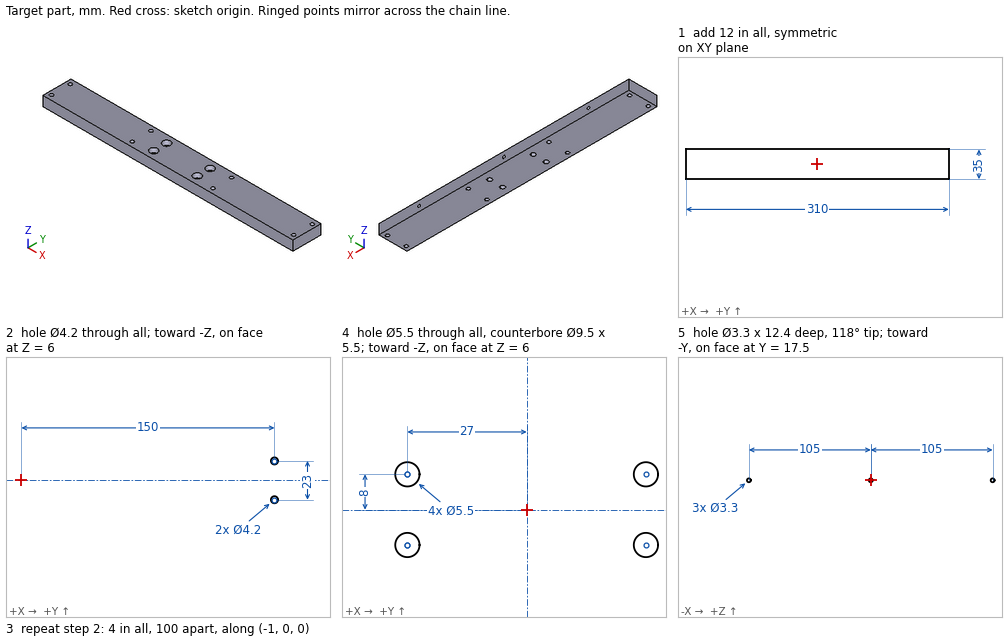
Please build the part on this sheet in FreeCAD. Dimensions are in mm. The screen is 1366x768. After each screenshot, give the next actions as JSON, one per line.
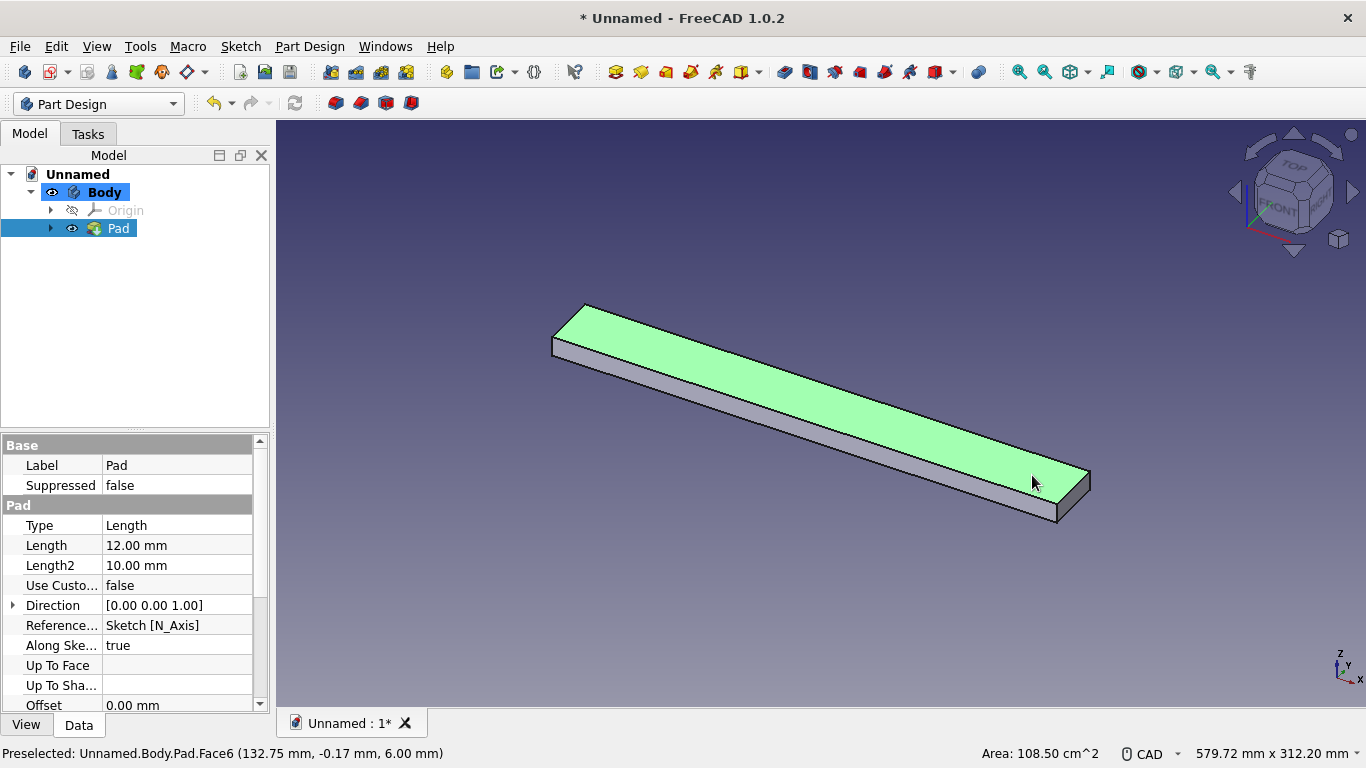
{"action": "left_click", "coordinate": [50, 72]}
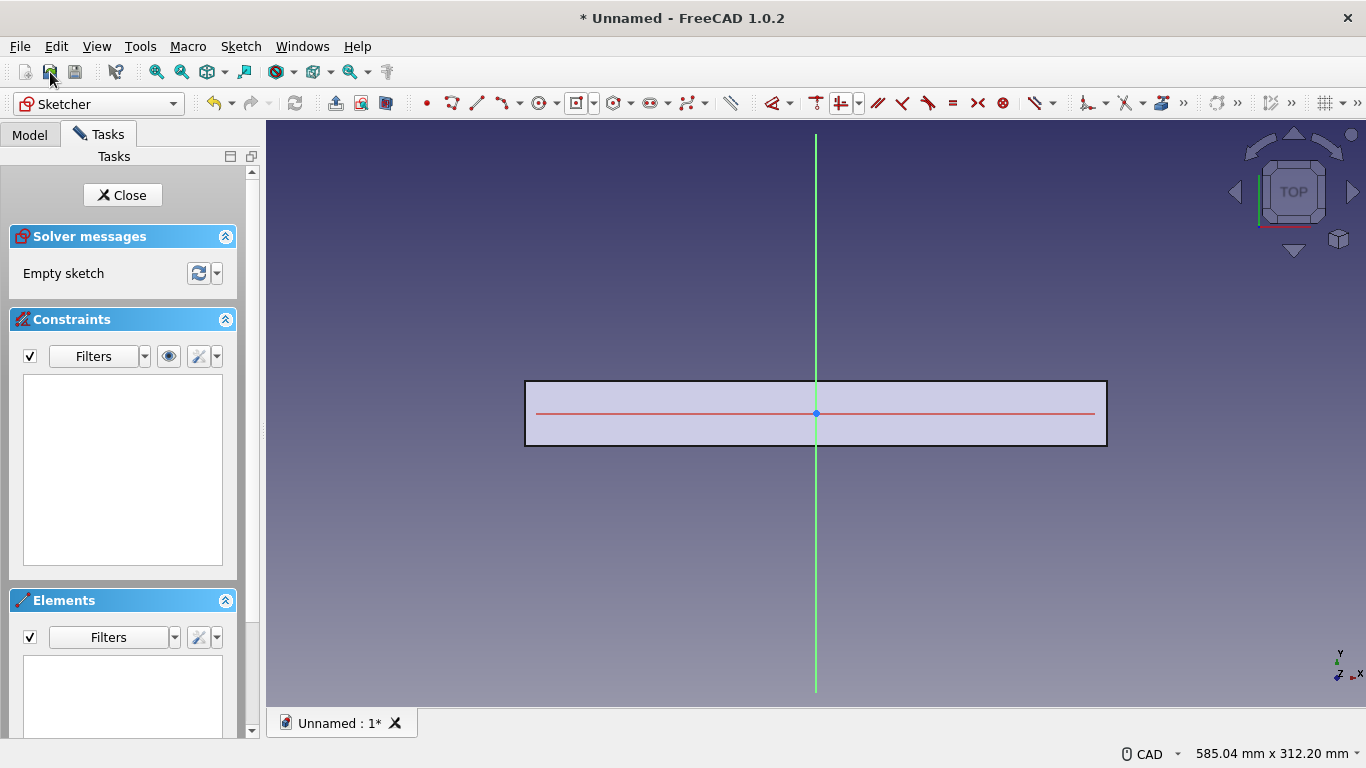
{"action": "scroll", "coordinate": [1153, 414], "scroll_direction": "up", "scroll_amount": 10}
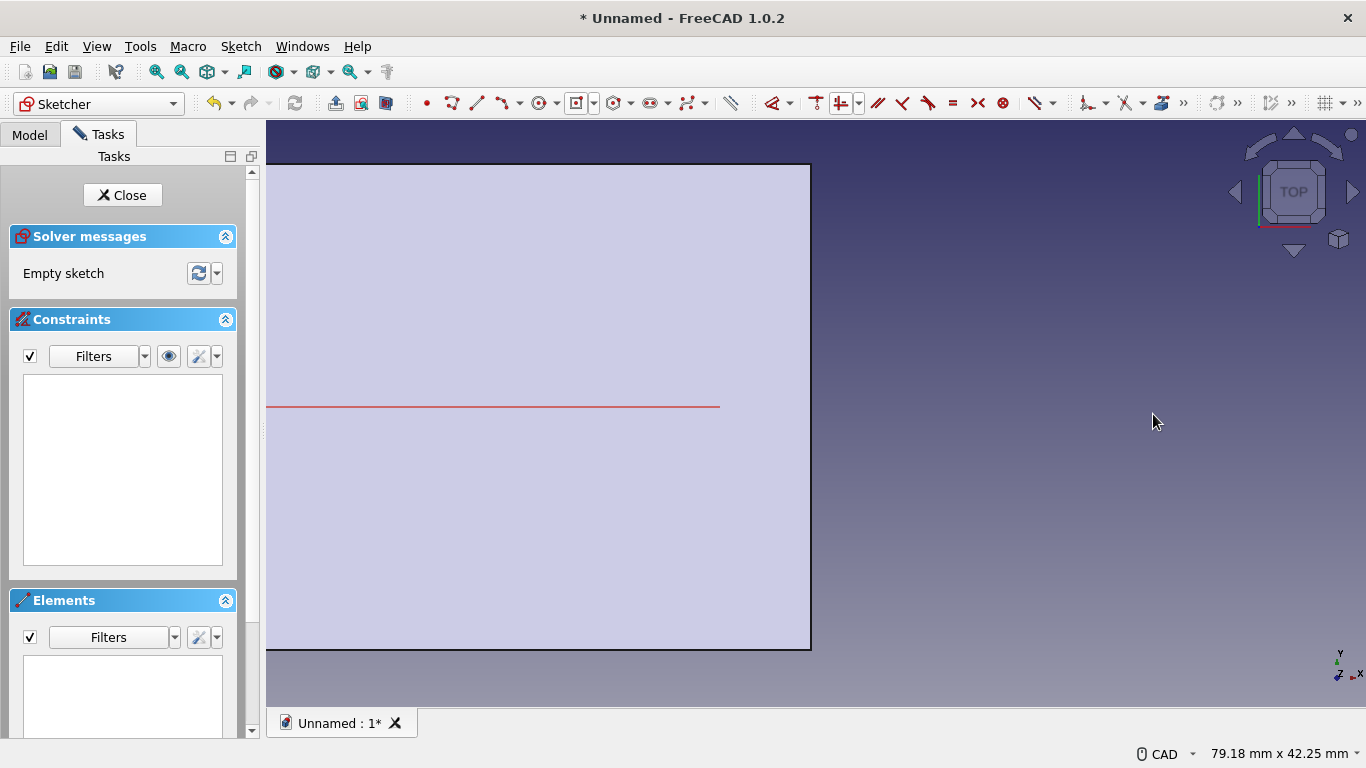
{"action": "left_click", "coordinate": [538, 104]}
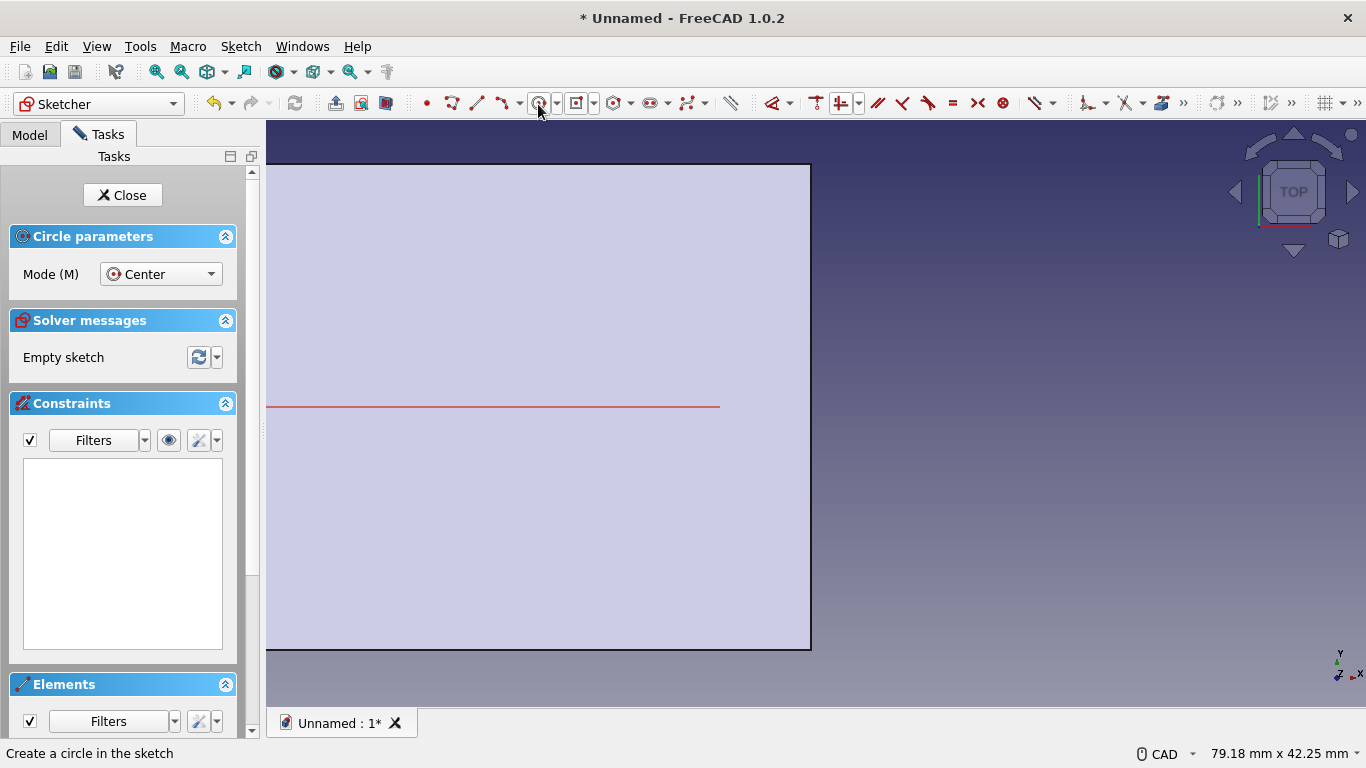
{"action": "left_click", "coordinate": [742, 247]}
{"action": "left_click", "coordinate": [762, 227]}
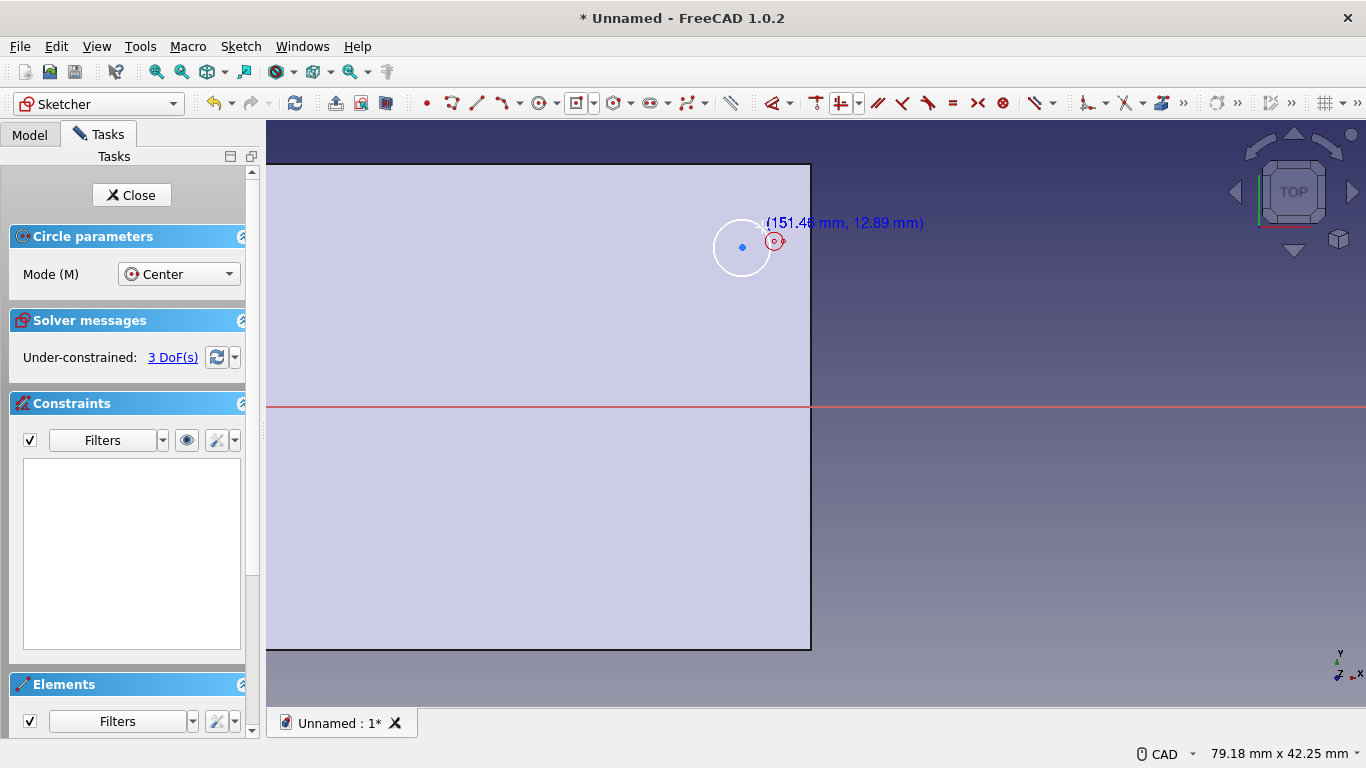
{"action": "left_click", "coordinate": [742, 567]}
{"action": "left_click", "coordinate": [762, 546]}
{"action": "key", "text": "Escape"}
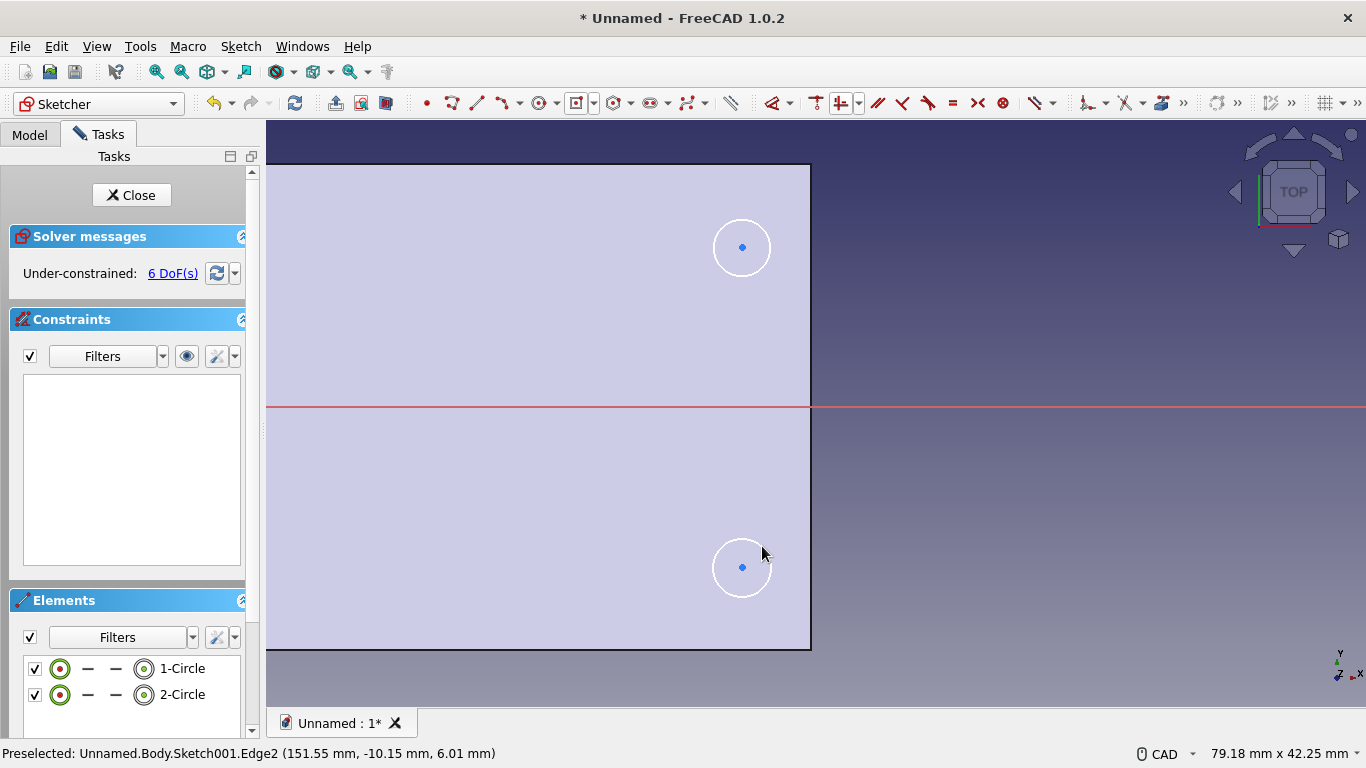
{"action": "left_click", "coordinate": [762, 228]}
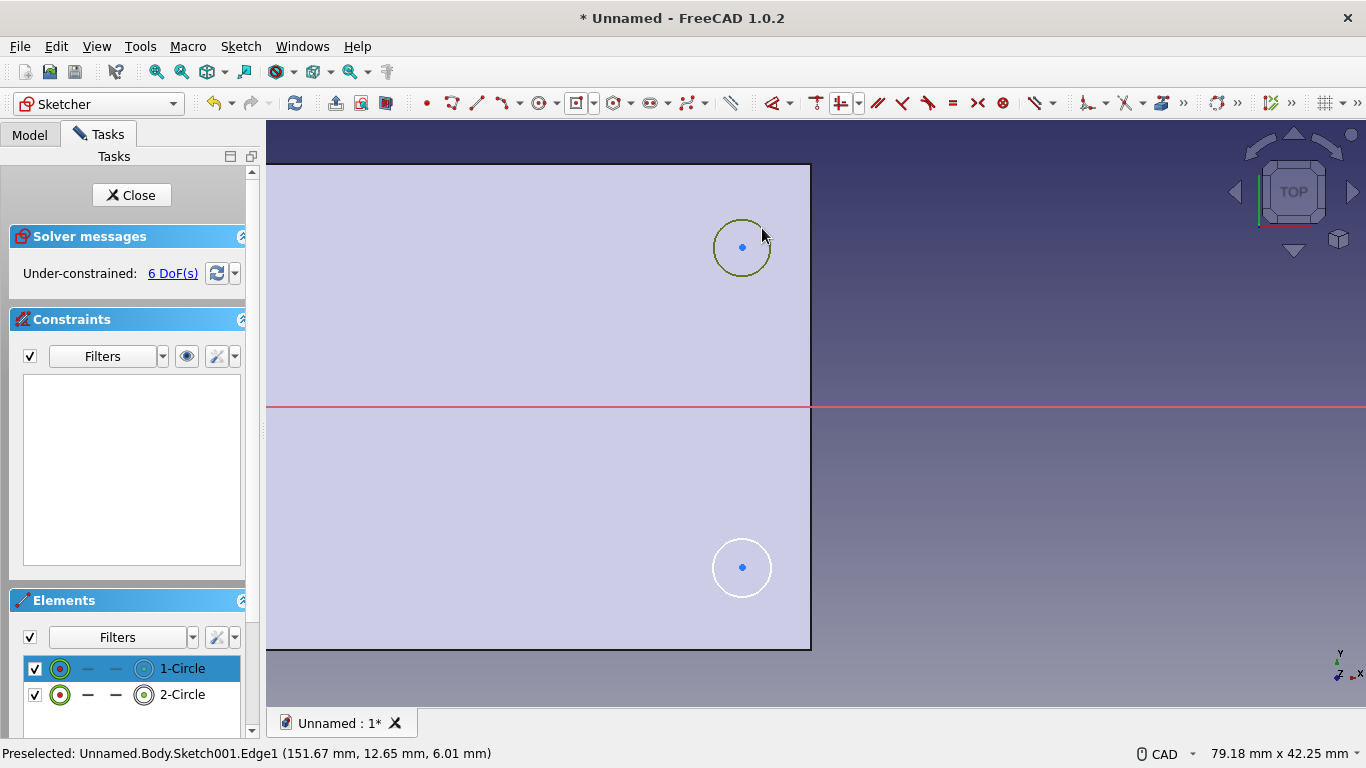
{"action": "left_click", "coordinate": [762, 547]}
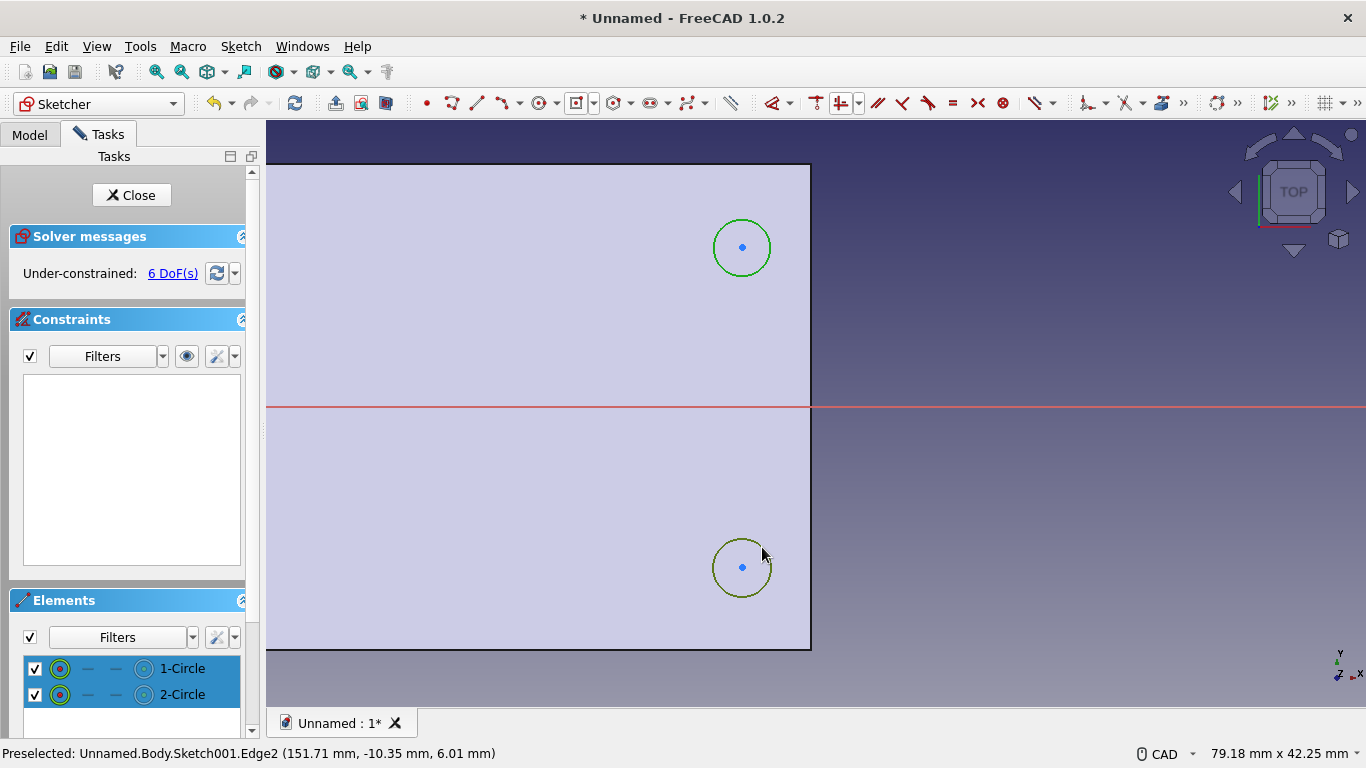
{"action": "left_click", "coordinate": [953, 104]}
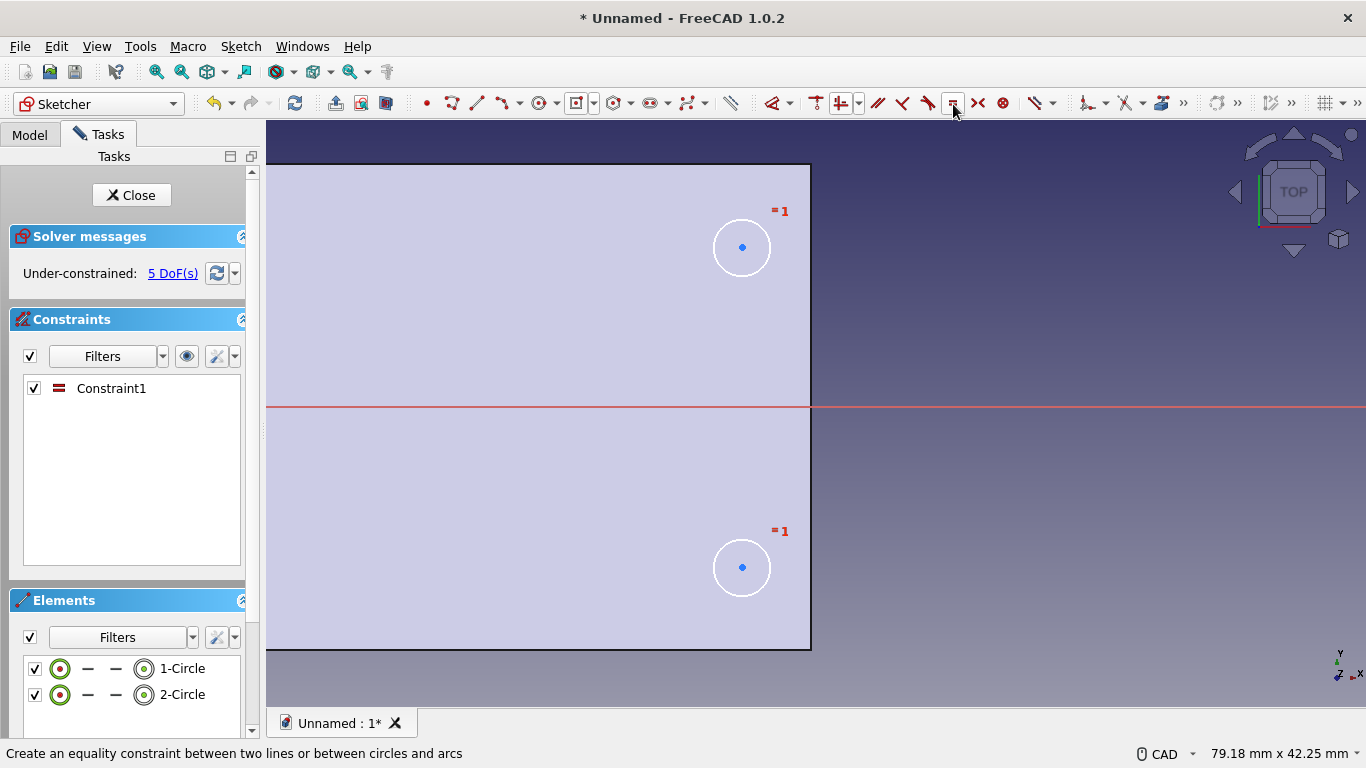
{"action": "left_click", "coordinate": [742, 248]}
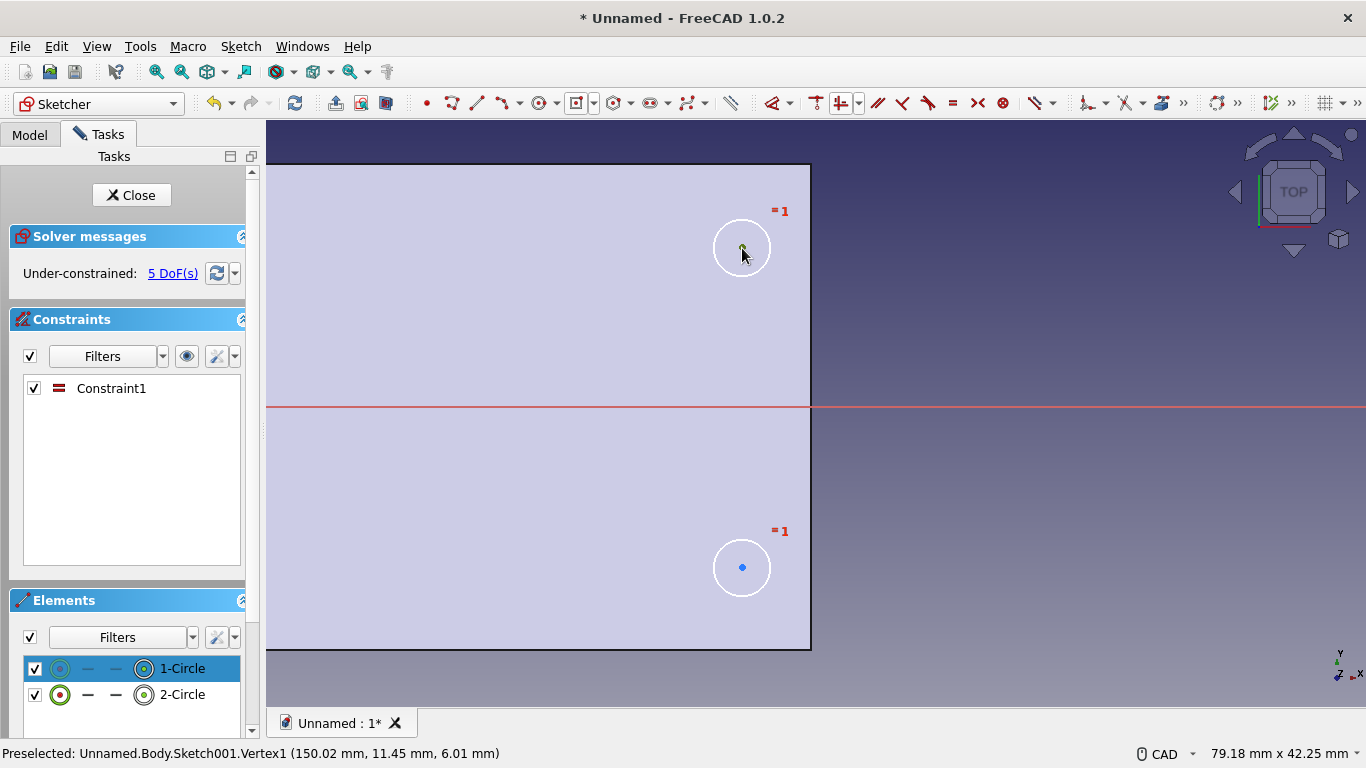
{"action": "left_click", "coordinate": [742, 568]}